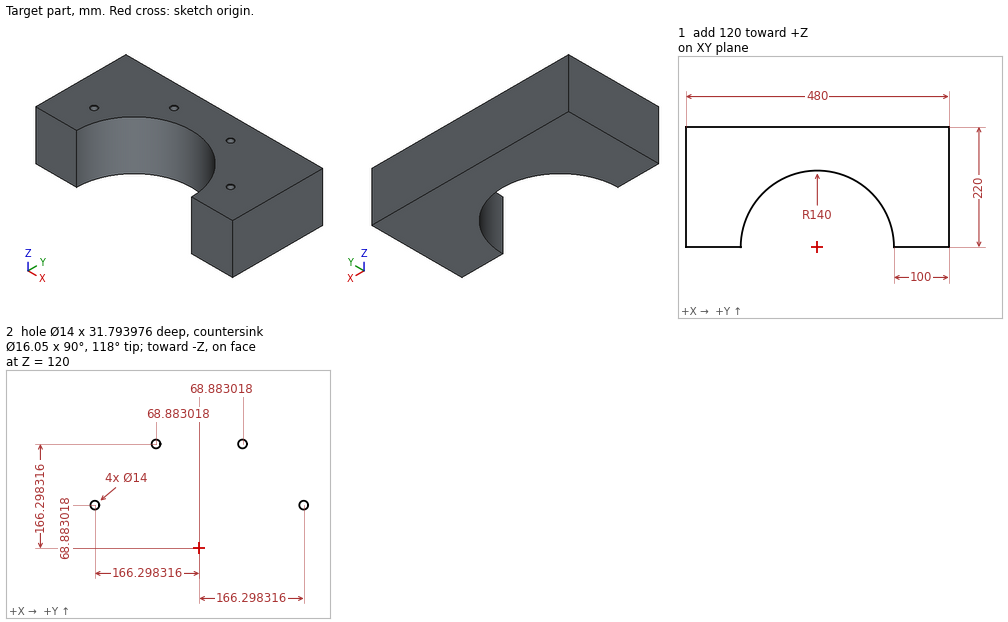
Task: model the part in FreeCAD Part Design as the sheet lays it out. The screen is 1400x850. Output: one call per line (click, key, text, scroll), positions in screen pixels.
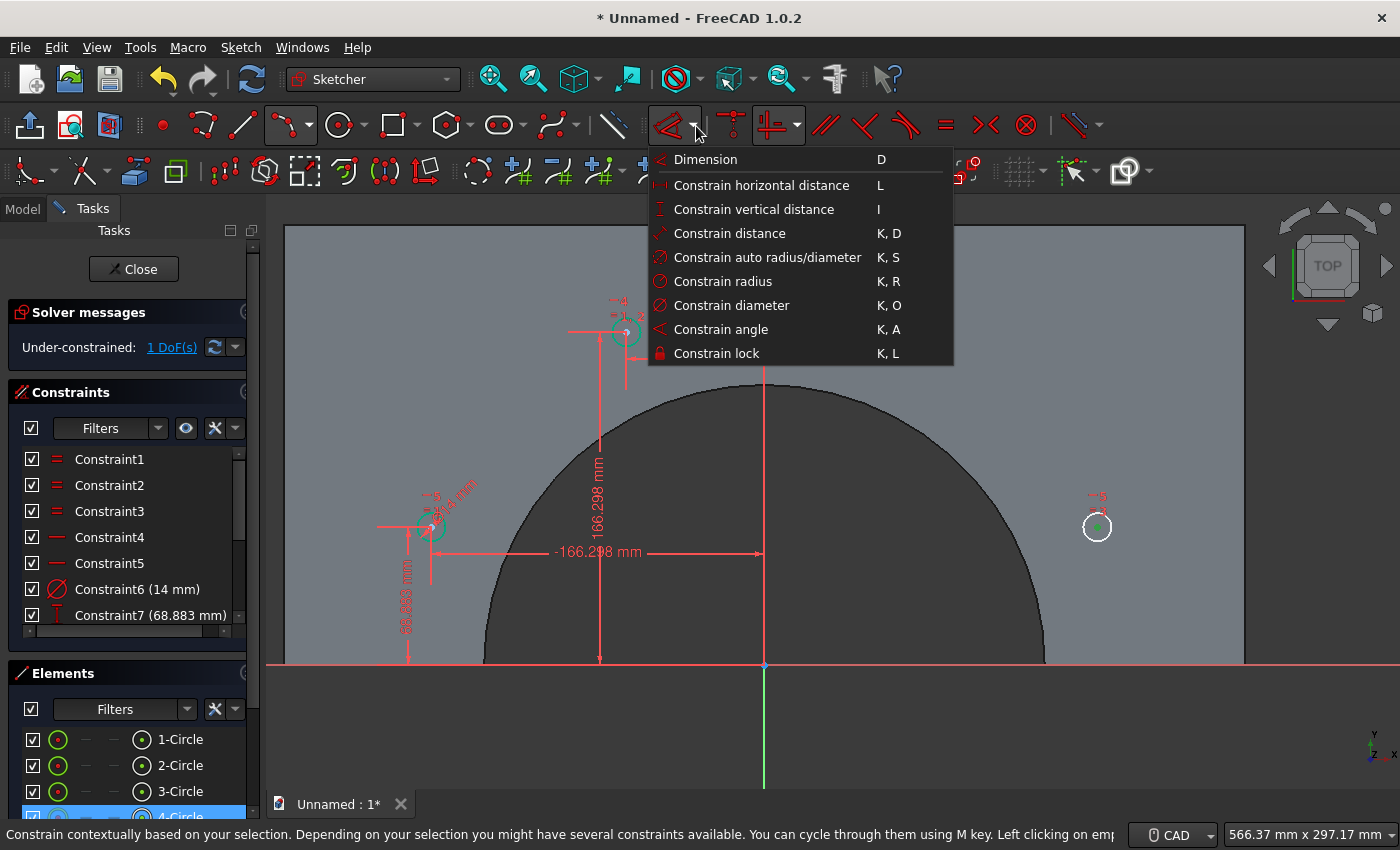
click(801, 185)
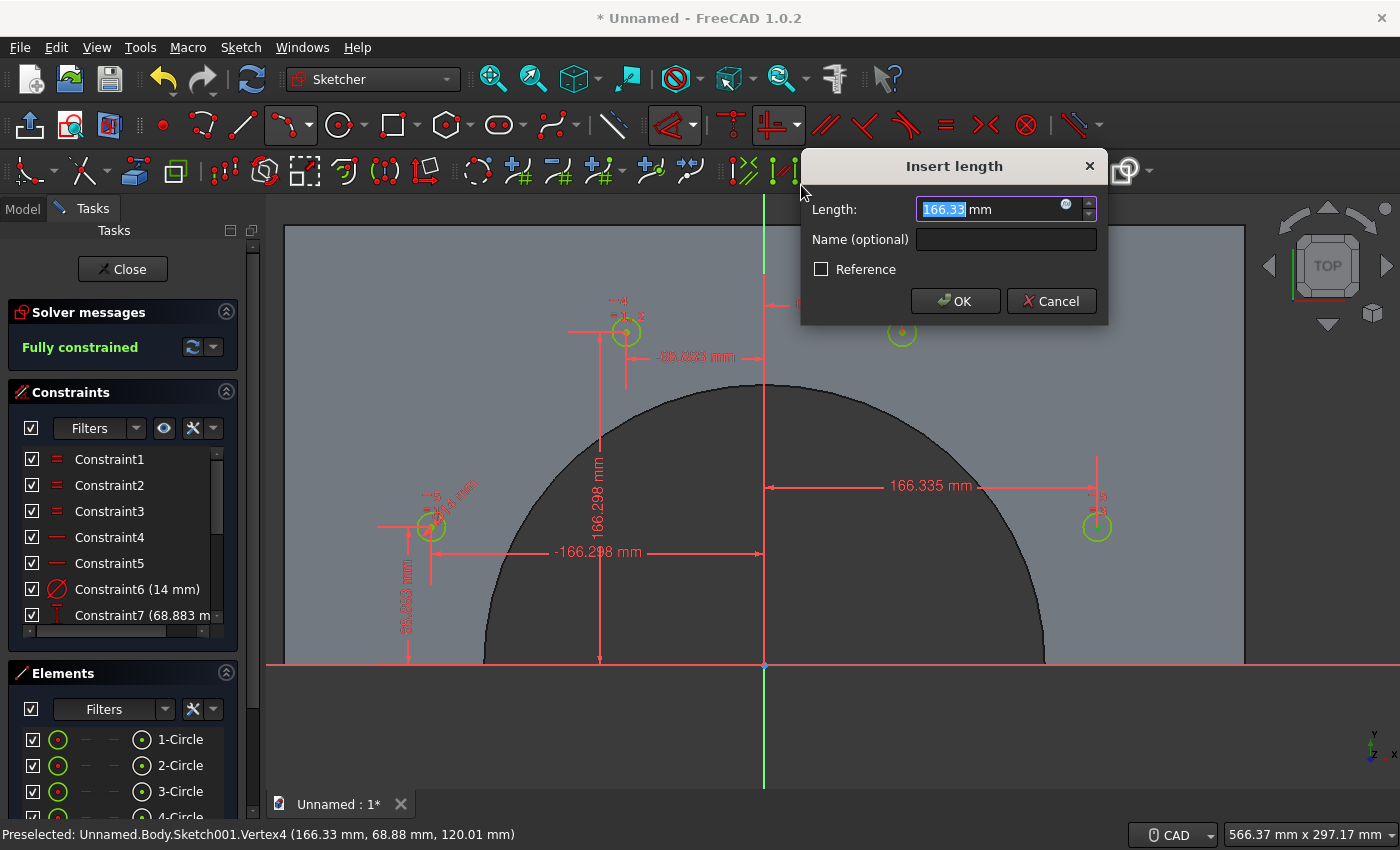
text(166.298316)
key(Return)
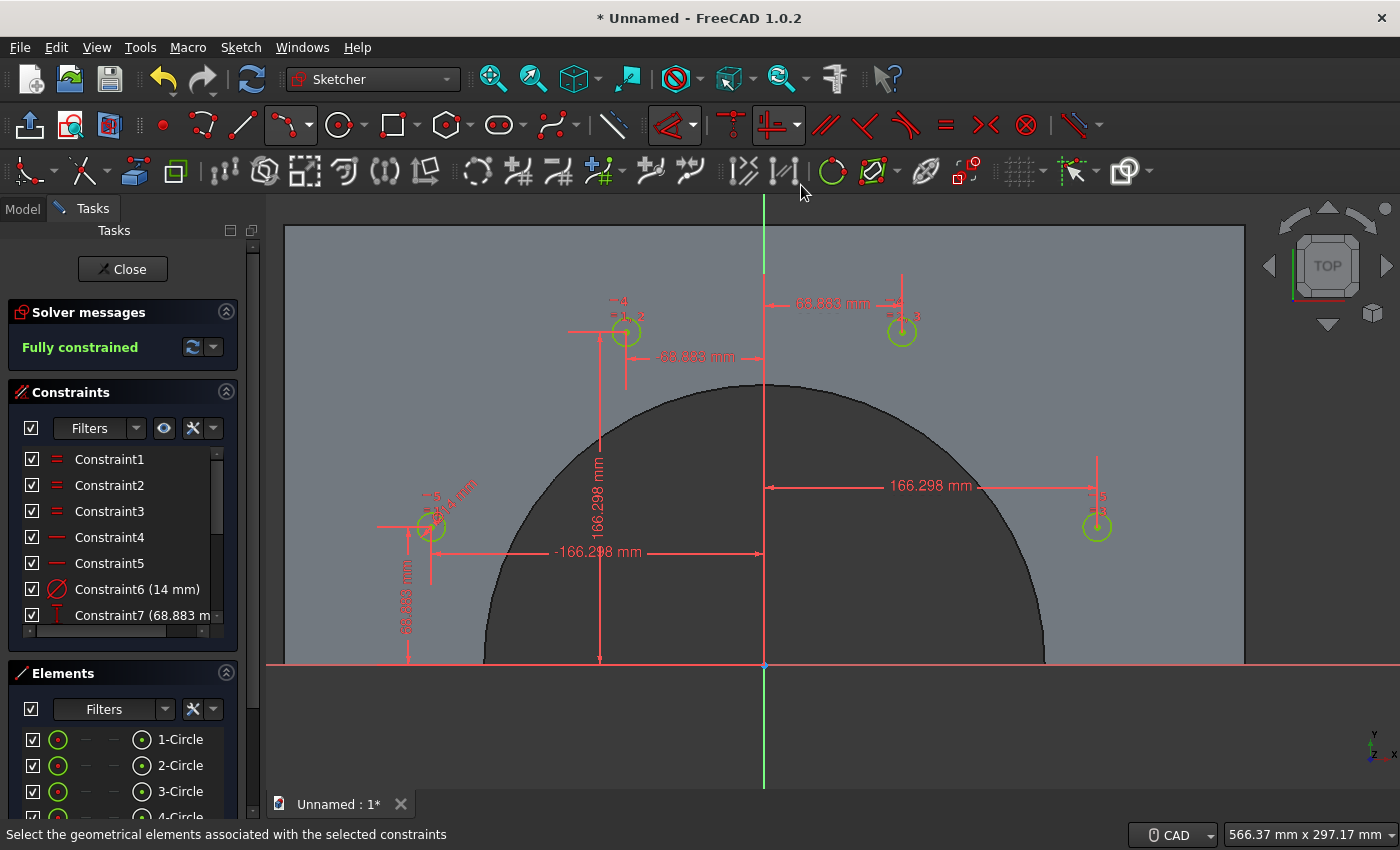
click(123, 269)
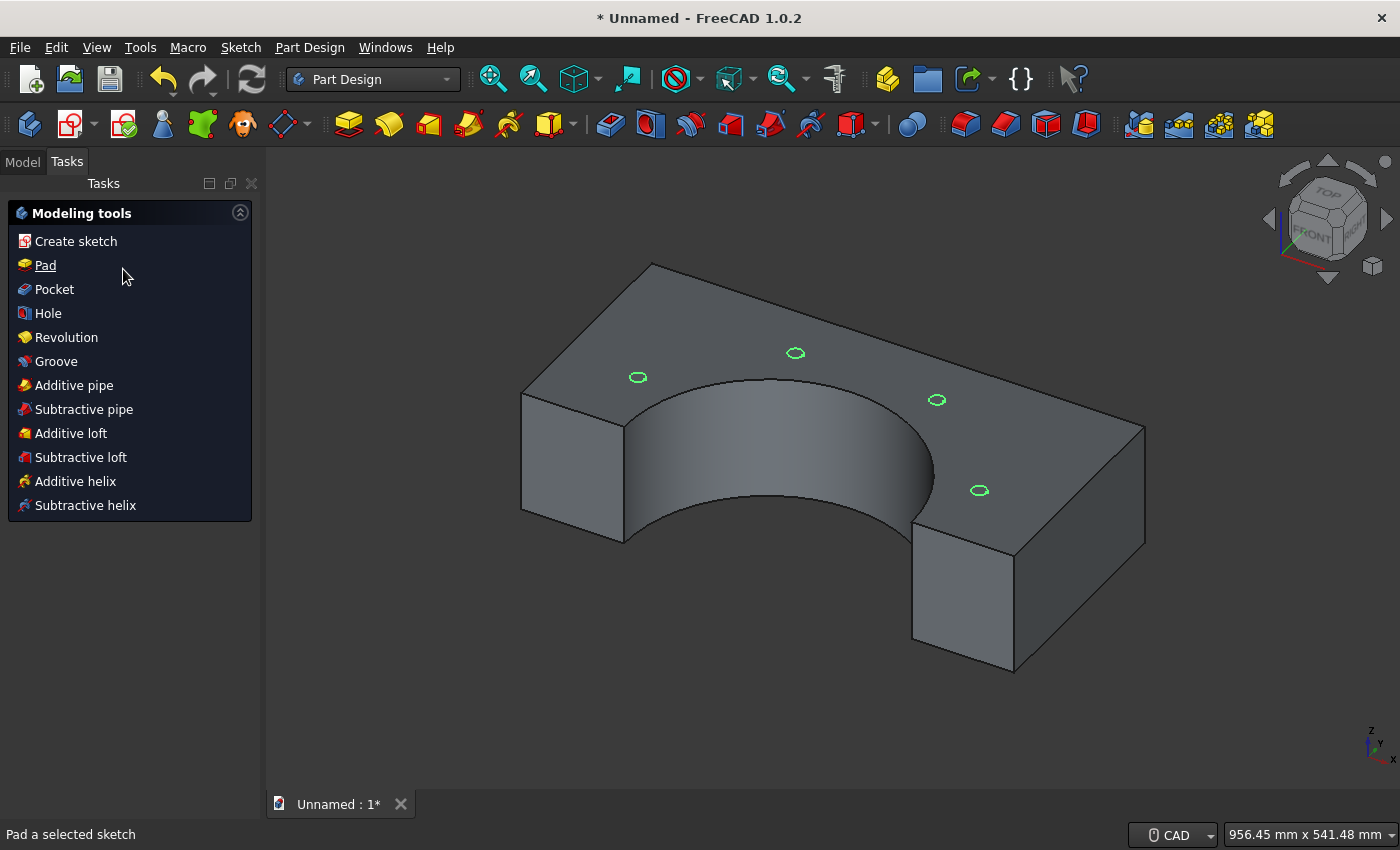
click(652, 124)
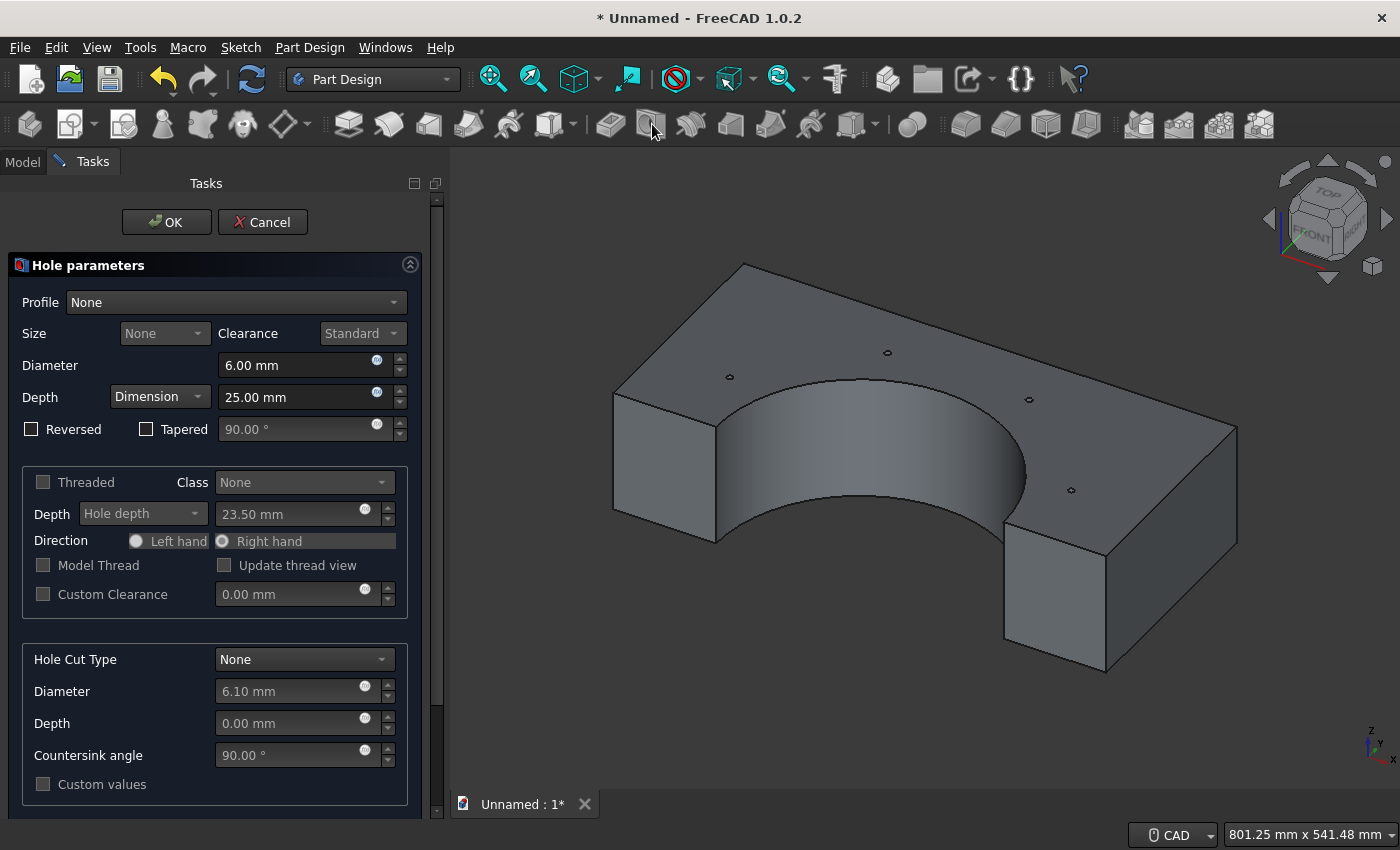
triple_click(305, 365)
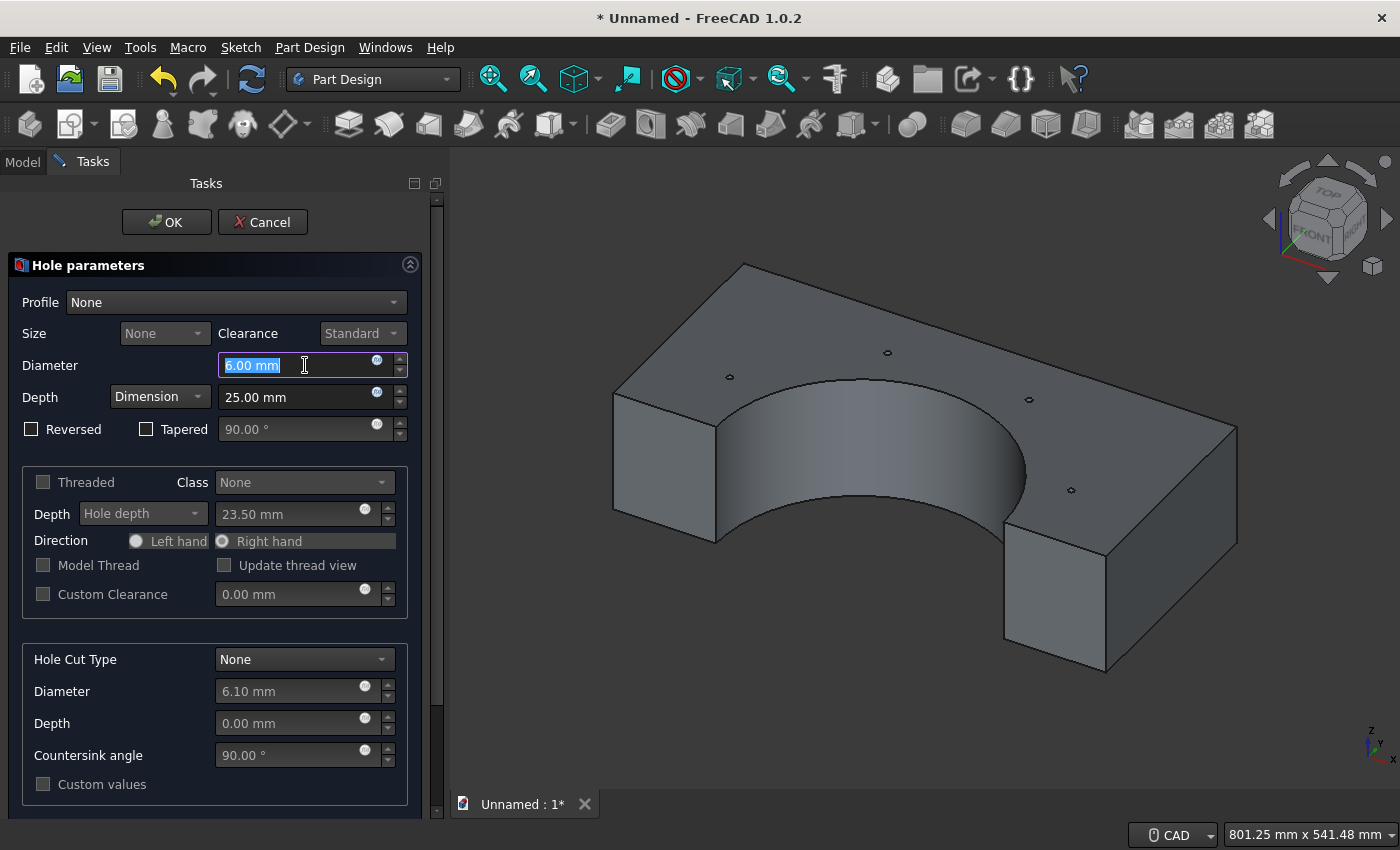
text(14)
key(Tab)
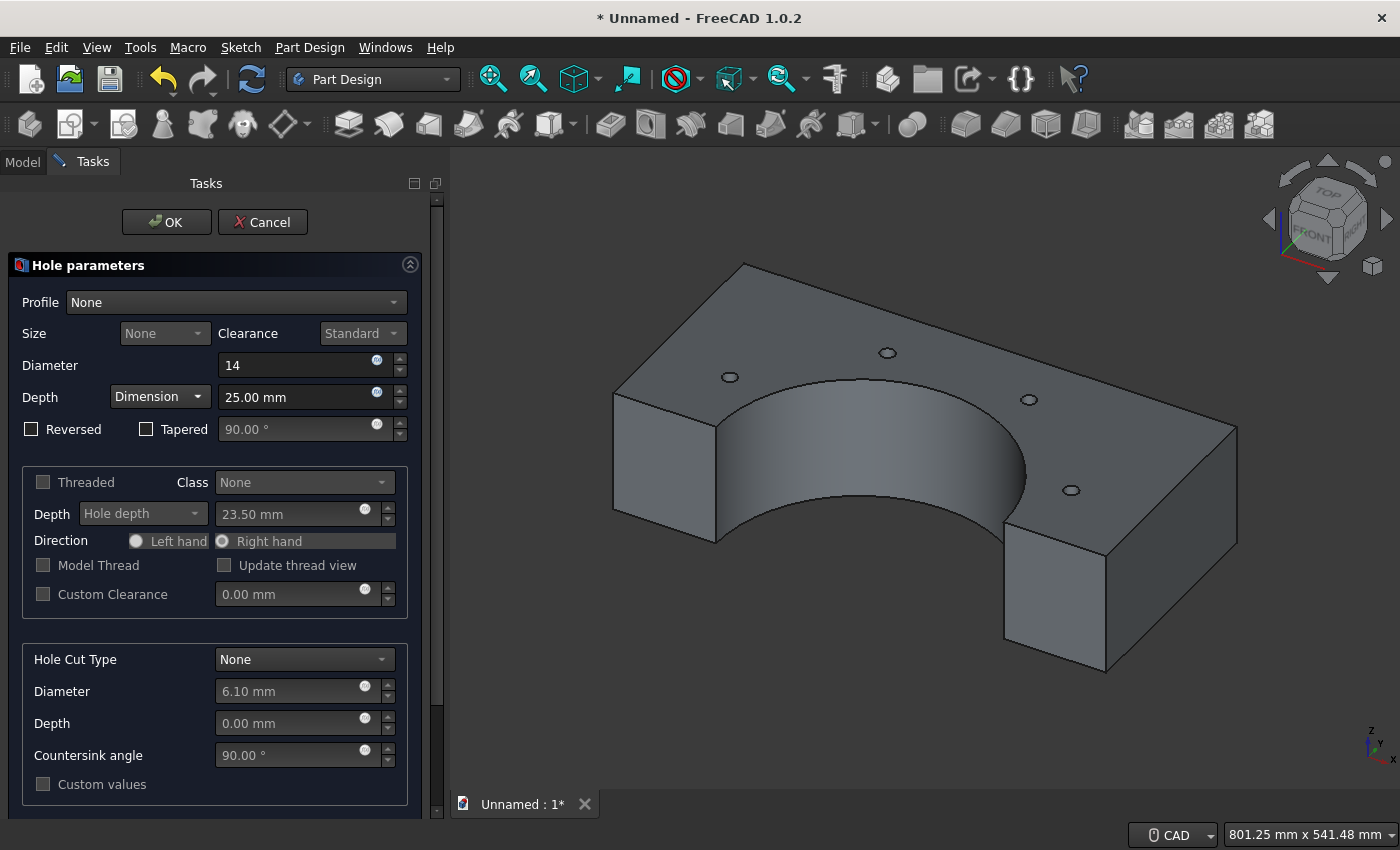
triple_click(305, 397)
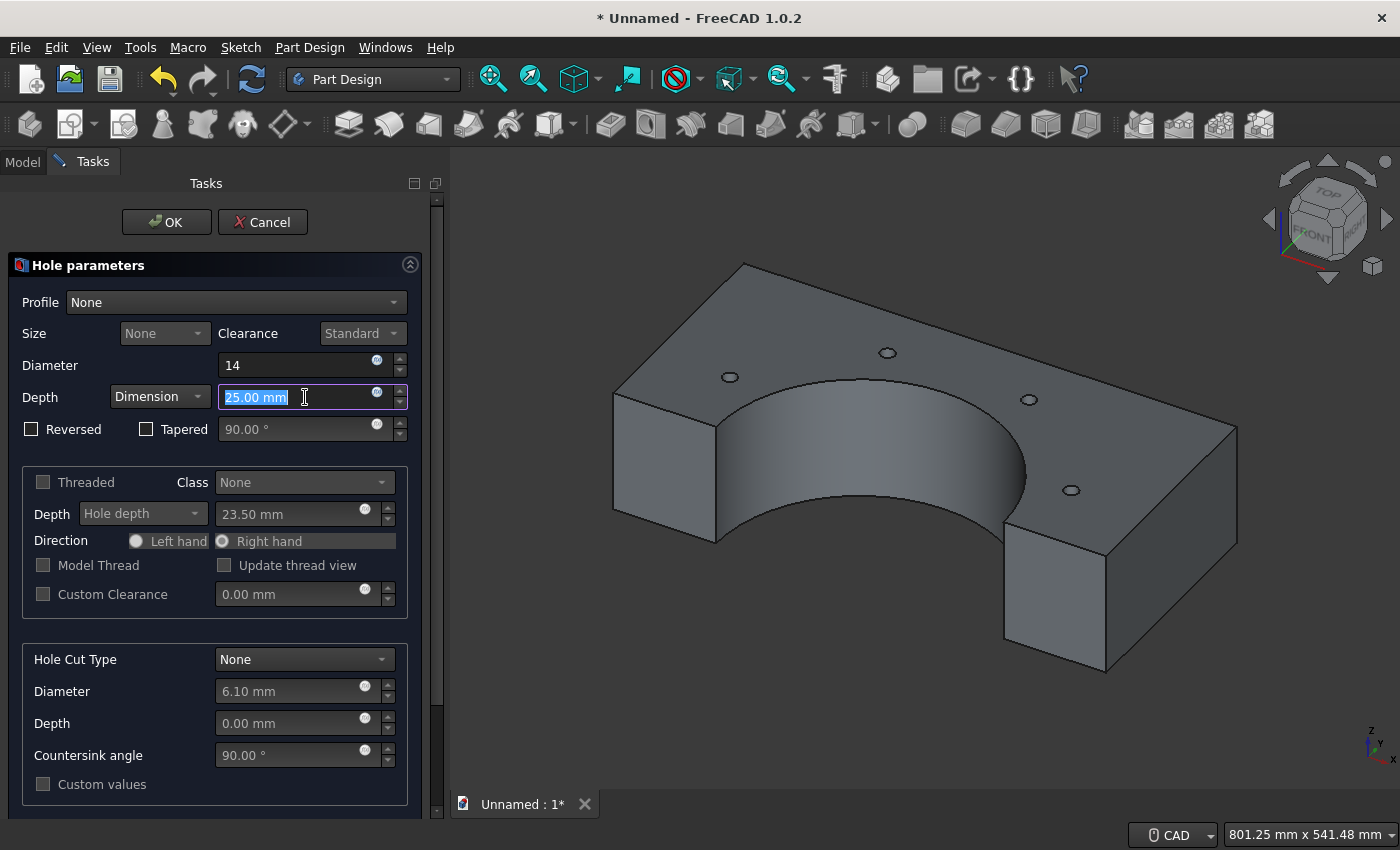
text(31.793976)
key(Tab)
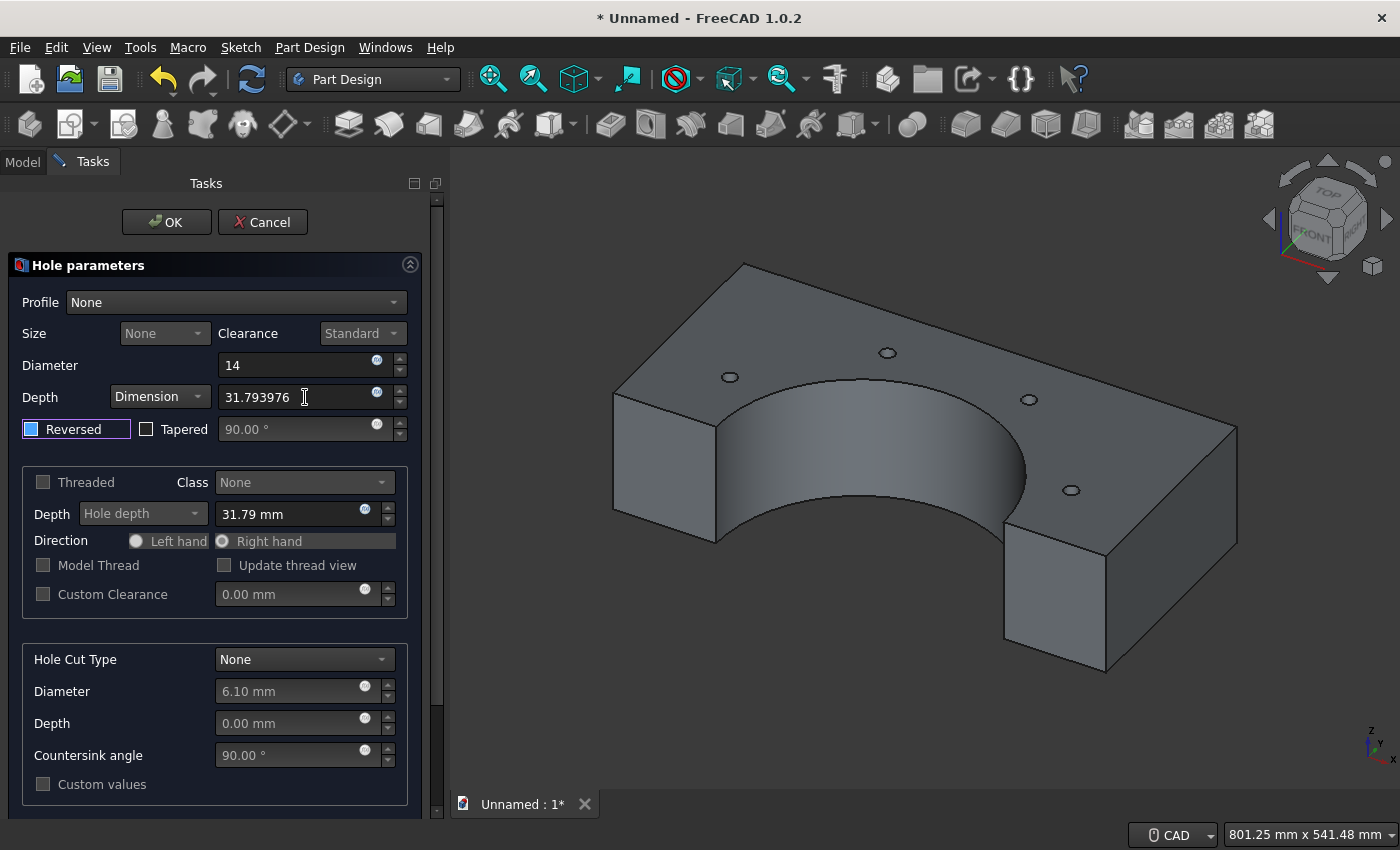
click(306, 660)